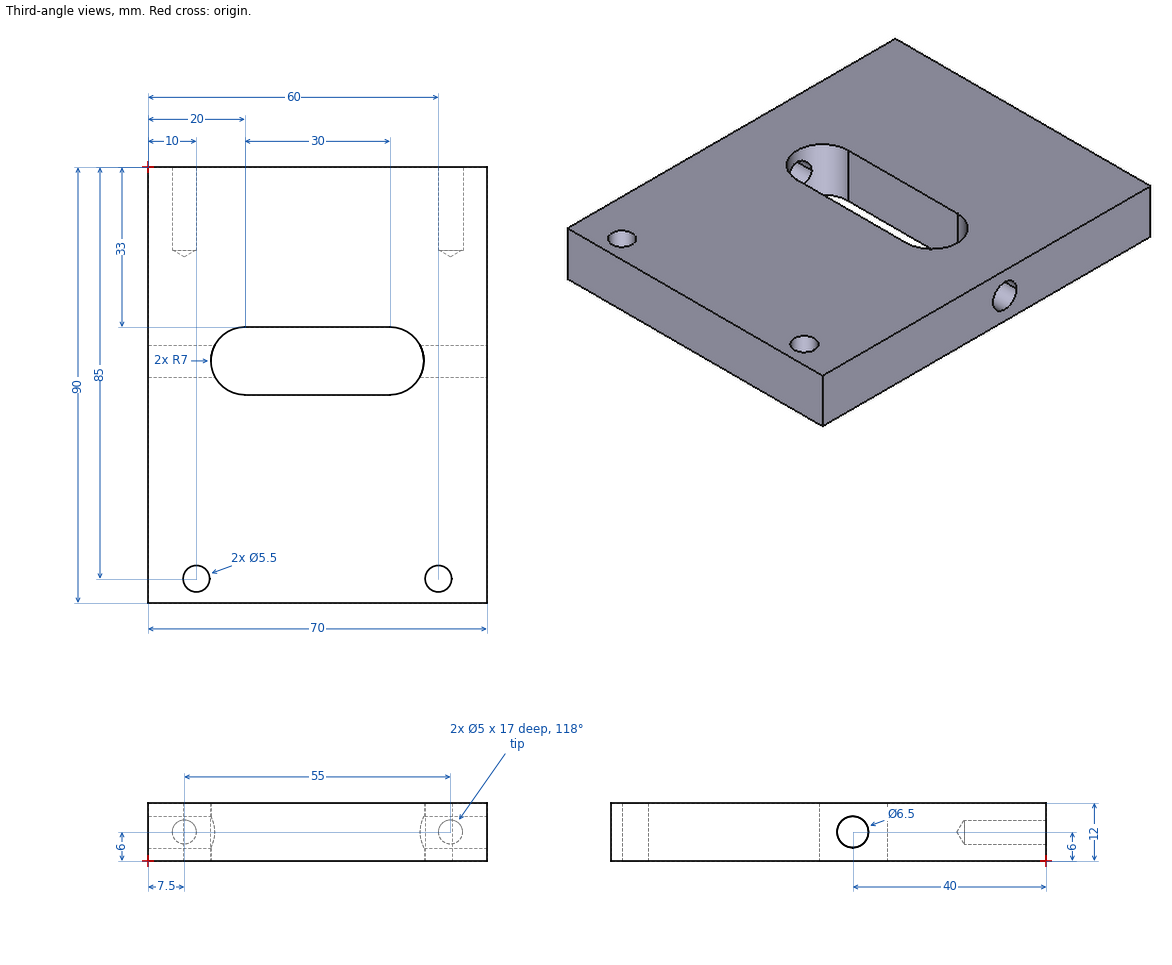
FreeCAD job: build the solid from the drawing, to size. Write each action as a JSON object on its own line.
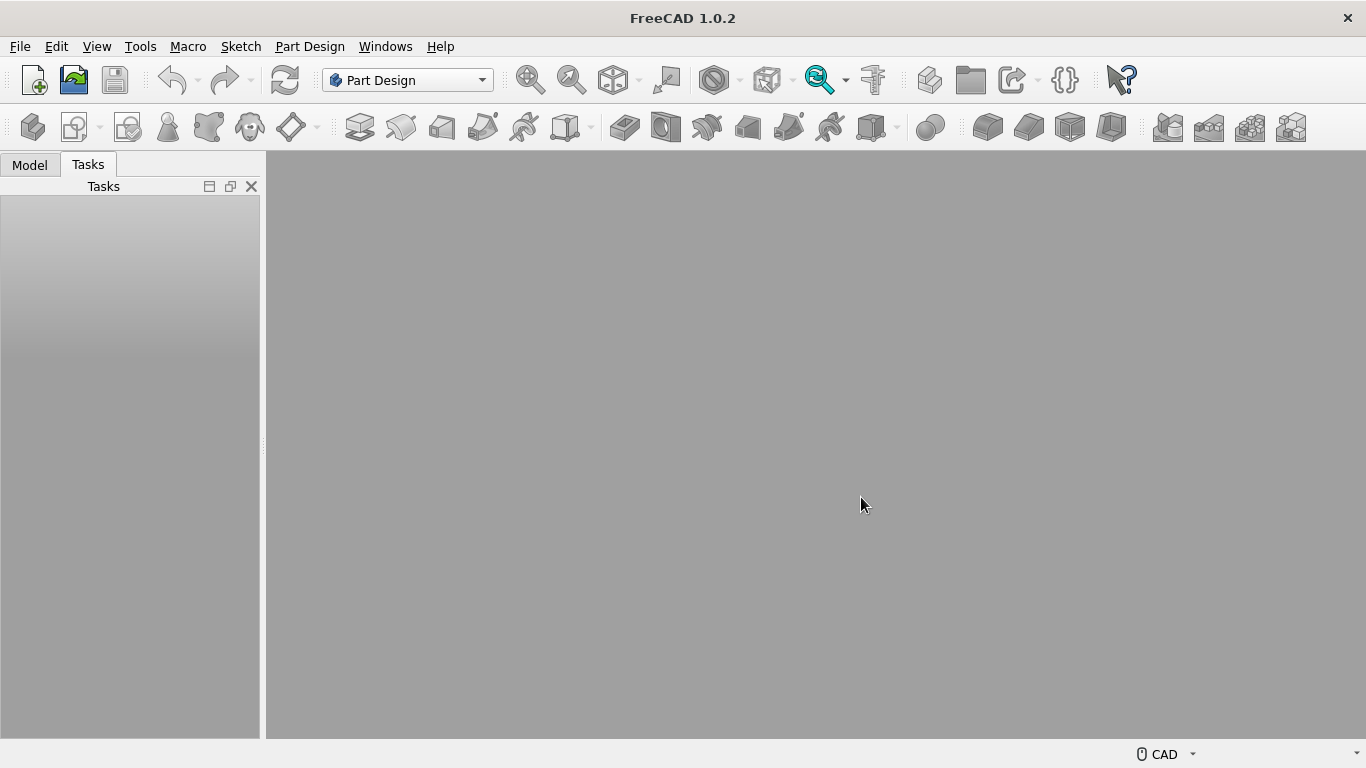
{"action": "left_click", "coordinate": [33, 80]}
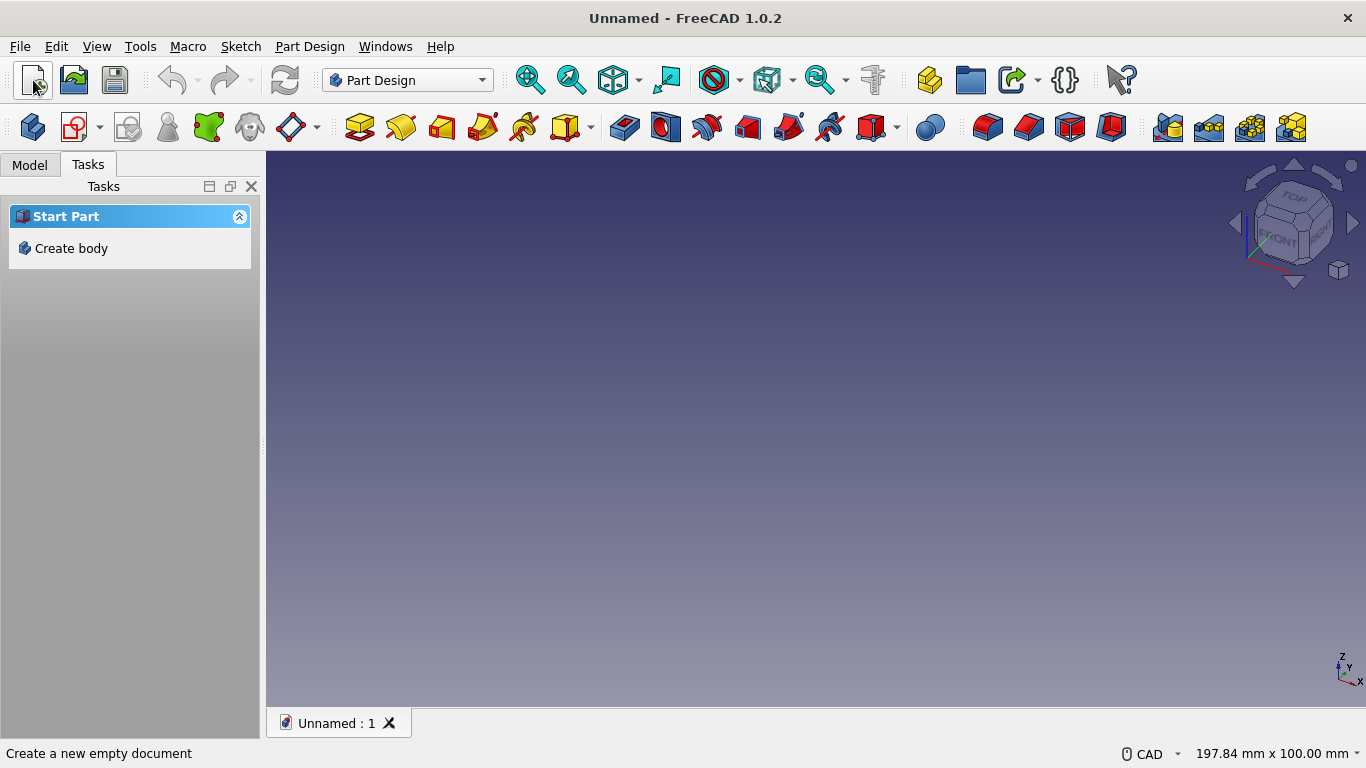
{"action": "left_click", "coordinate": [74, 128]}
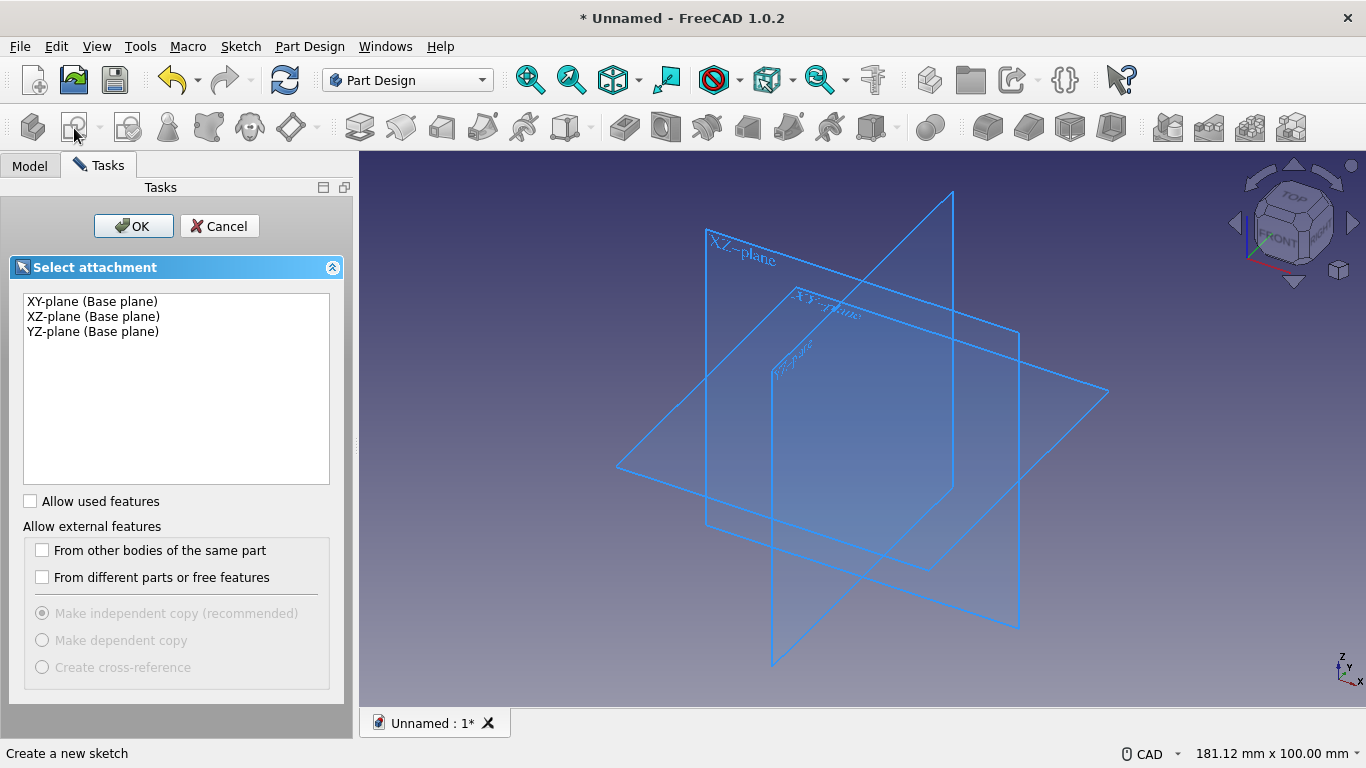
{"action": "left_click", "coordinate": [84, 302]}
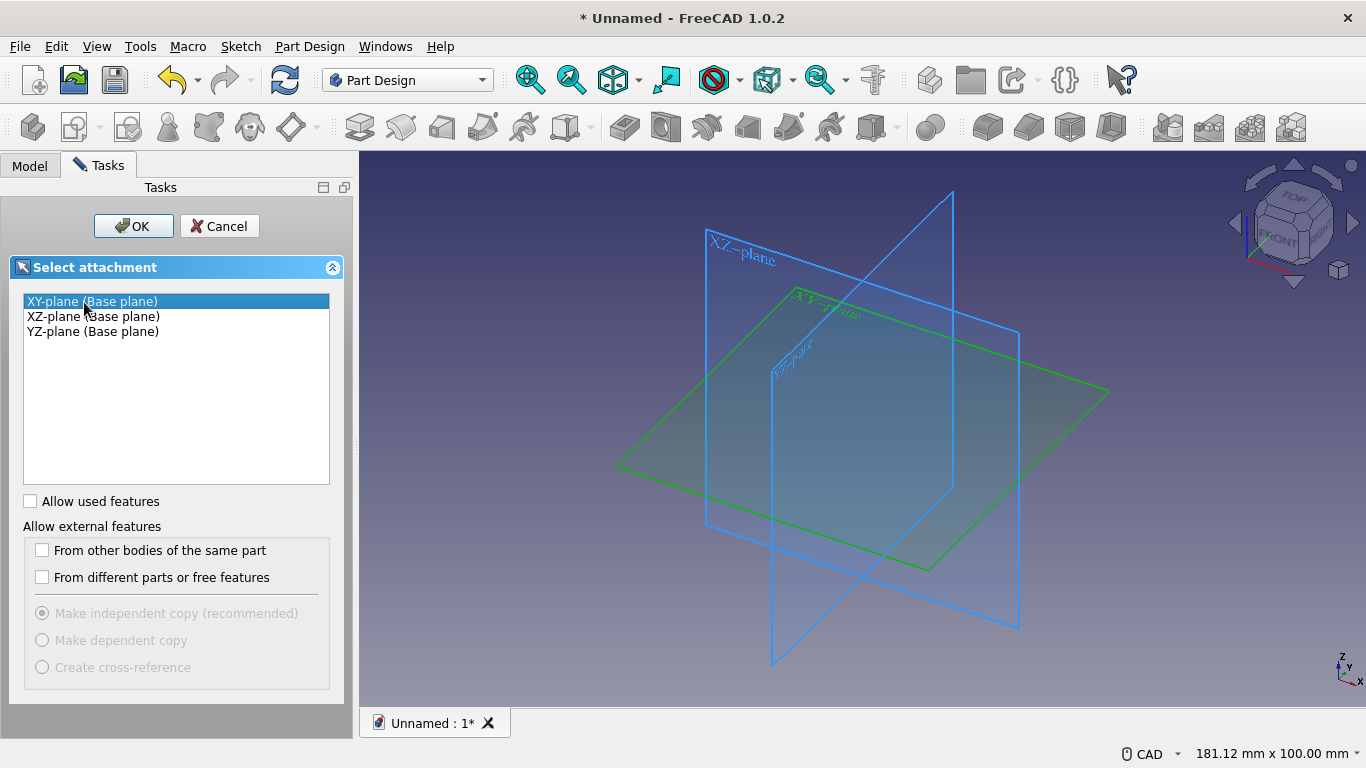
{"action": "left_click", "coordinate": [134, 226]}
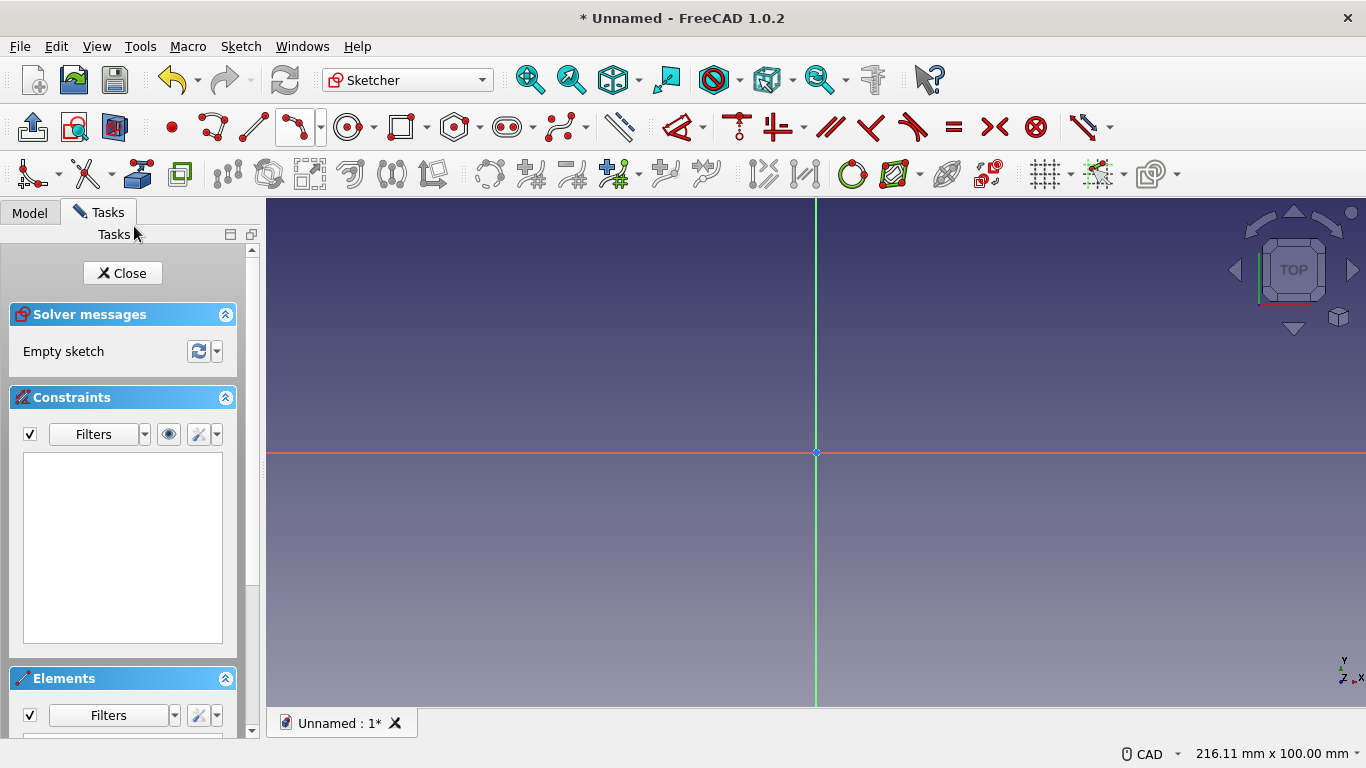
{"action": "scroll", "coordinate": [447, 226], "scroll_direction": "down", "scroll_amount": 3}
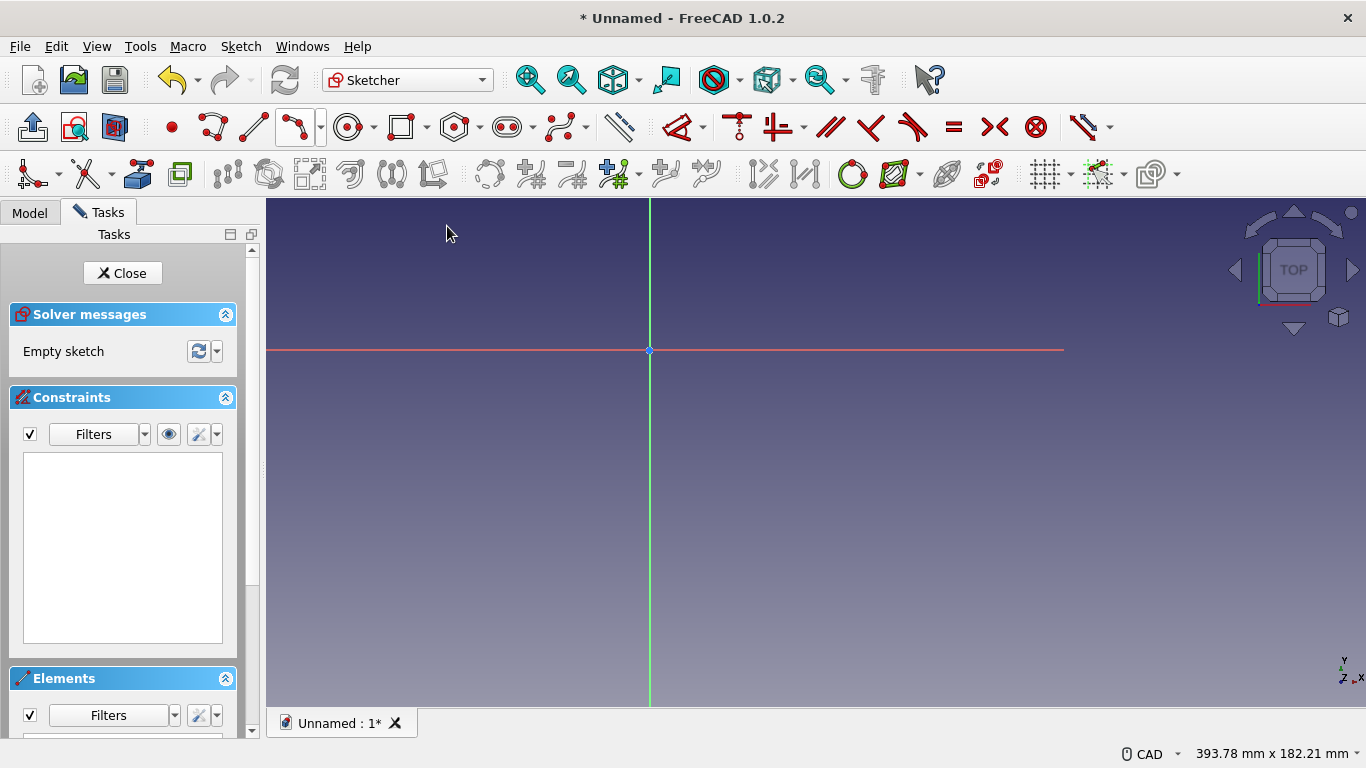
{"action": "left_click", "coordinate": [400, 128]}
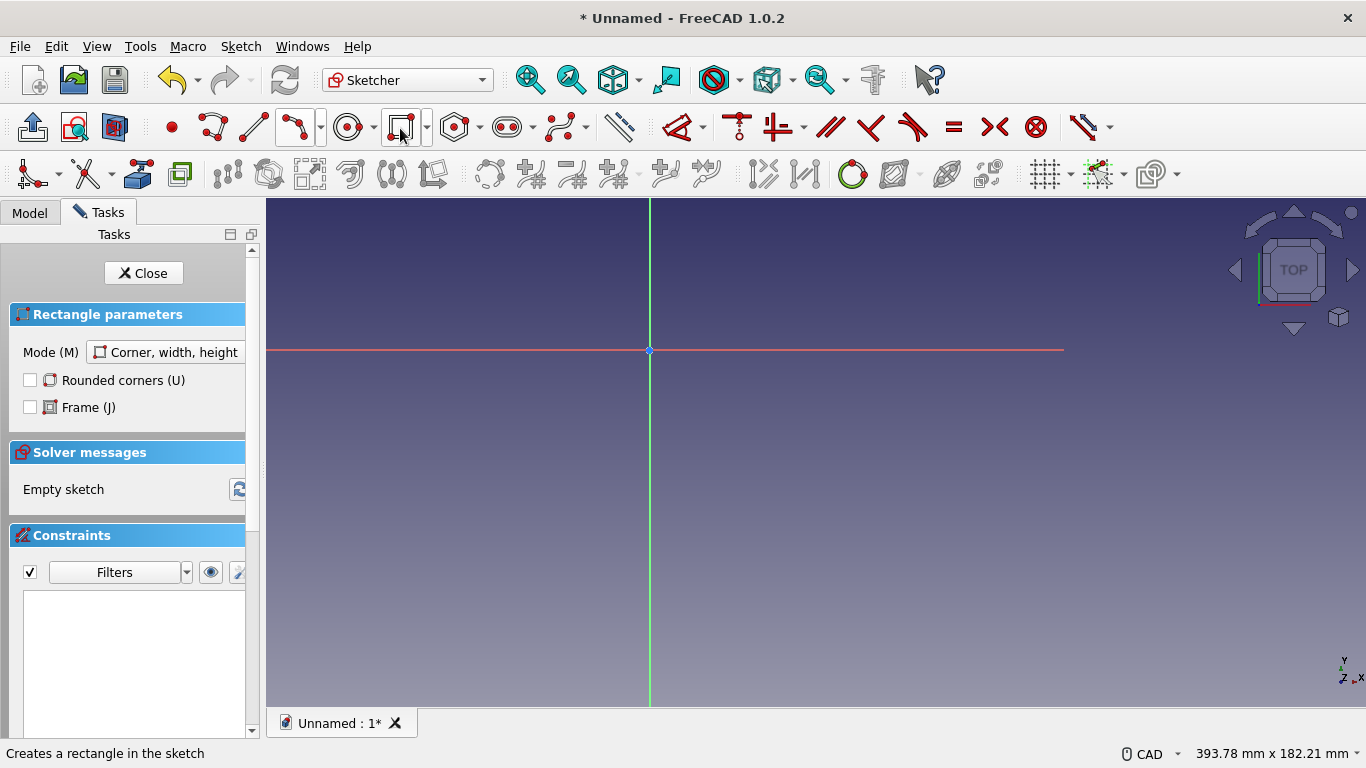
{"action": "left_click", "coordinate": [650, 350]}
{"action": "left_click", "coordinate": [845, 602]}
{"action": "key", "text": "Escape"}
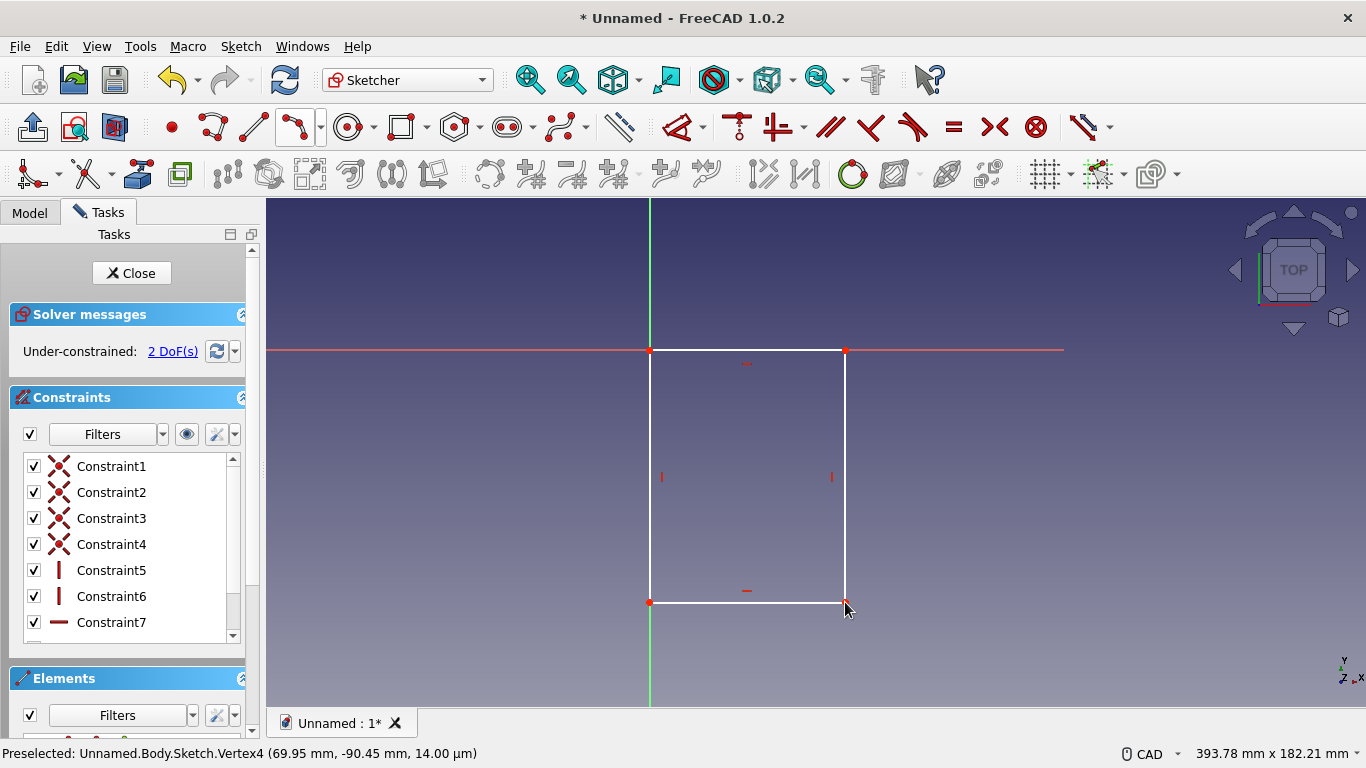
{"action": "left_click", "coordinate": [676, 128]}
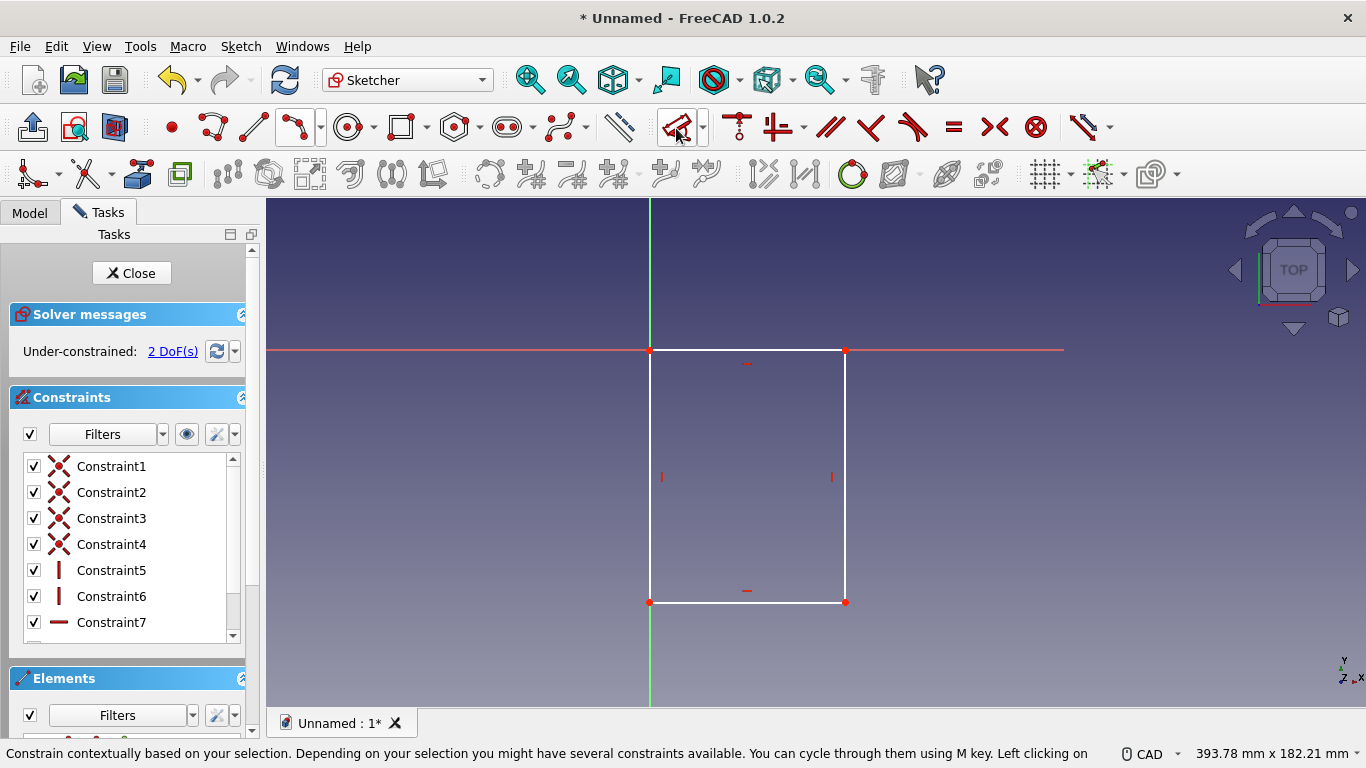
{"action": "left_click", "coordinate": [650, 426]}
{"action": "left_click", "coordinate": [616, 477]}